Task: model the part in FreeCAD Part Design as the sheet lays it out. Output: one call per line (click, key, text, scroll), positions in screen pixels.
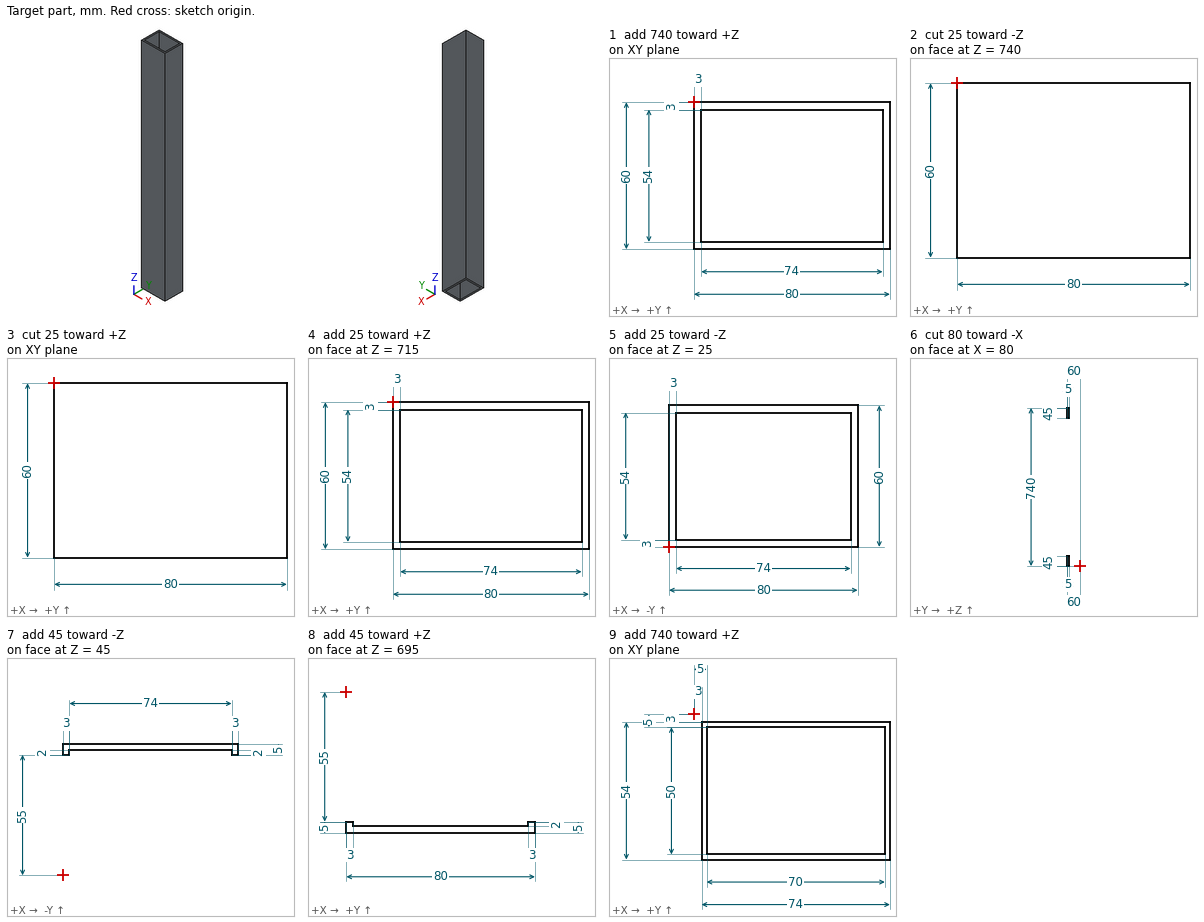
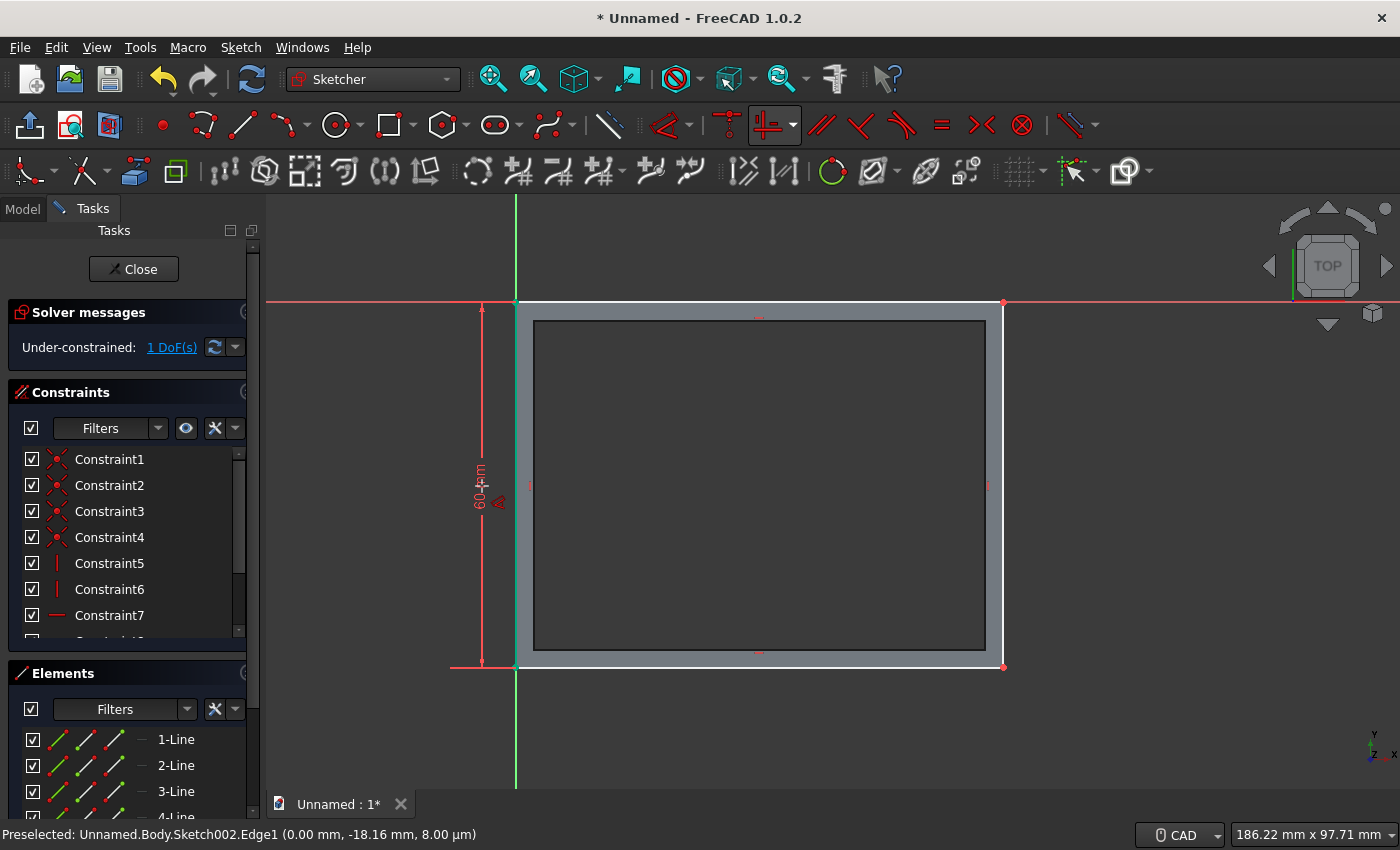
click(662, 668)
click(759, 702)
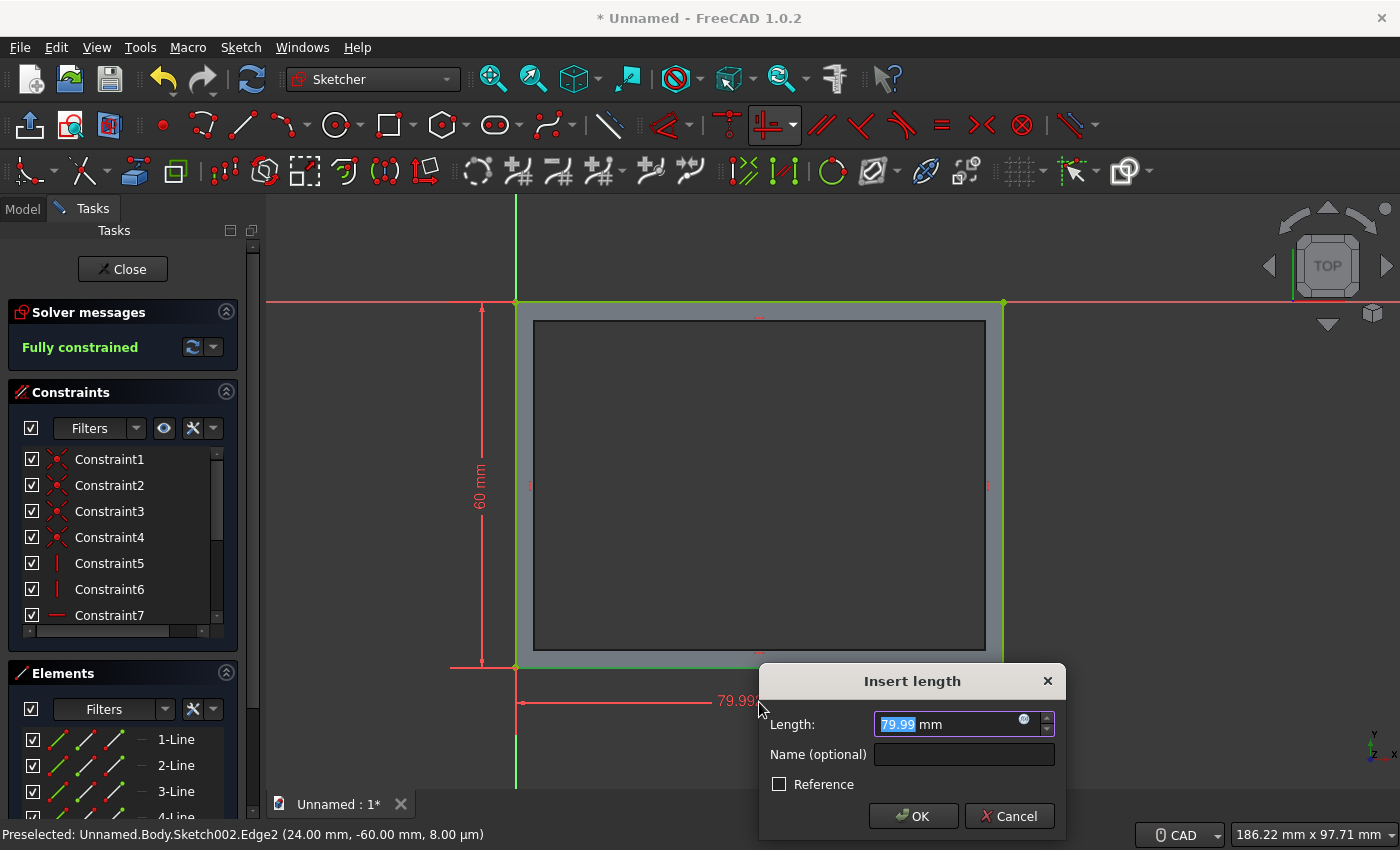
text(80)
key(Return)
key(Escape)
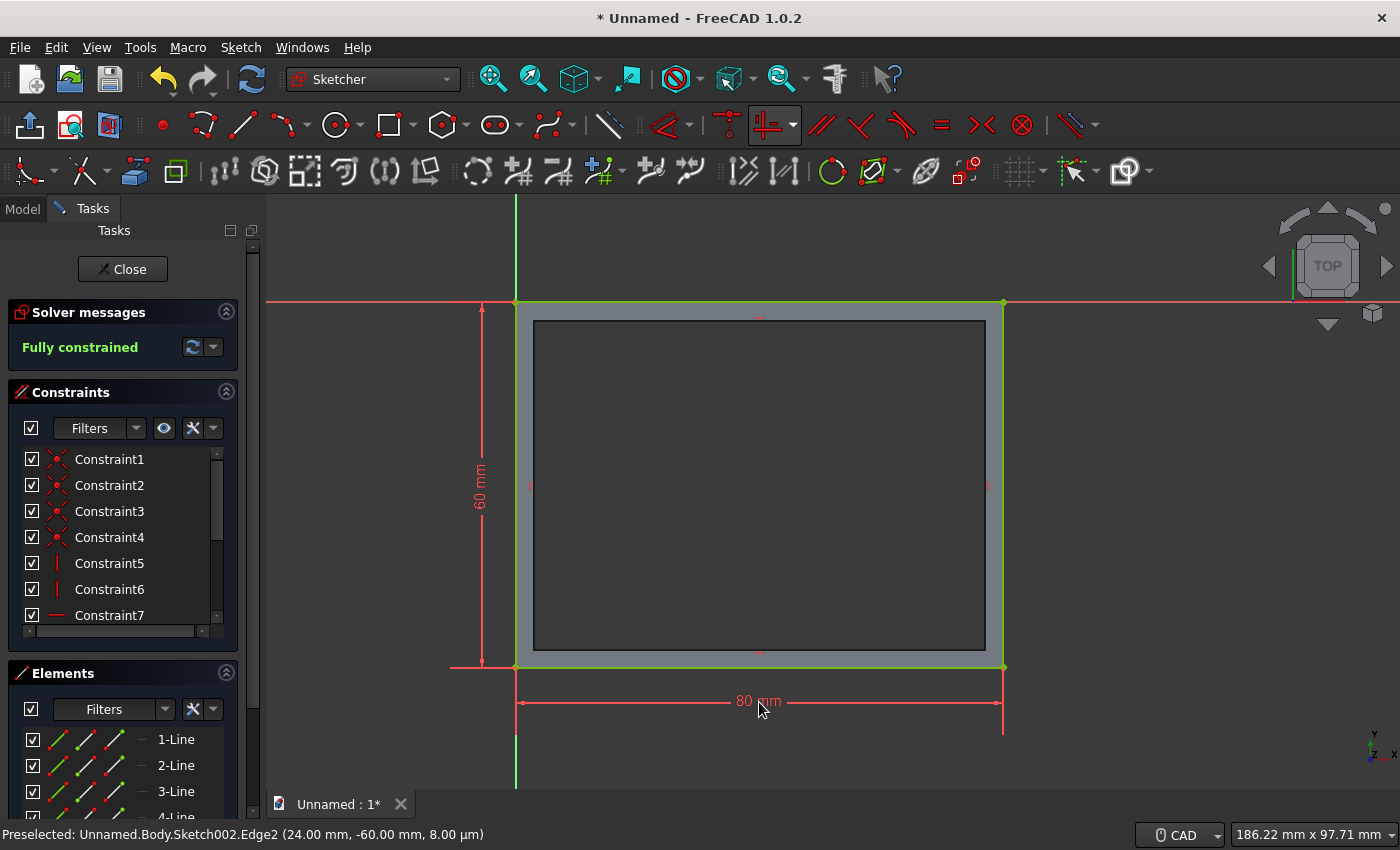
click(123, 269)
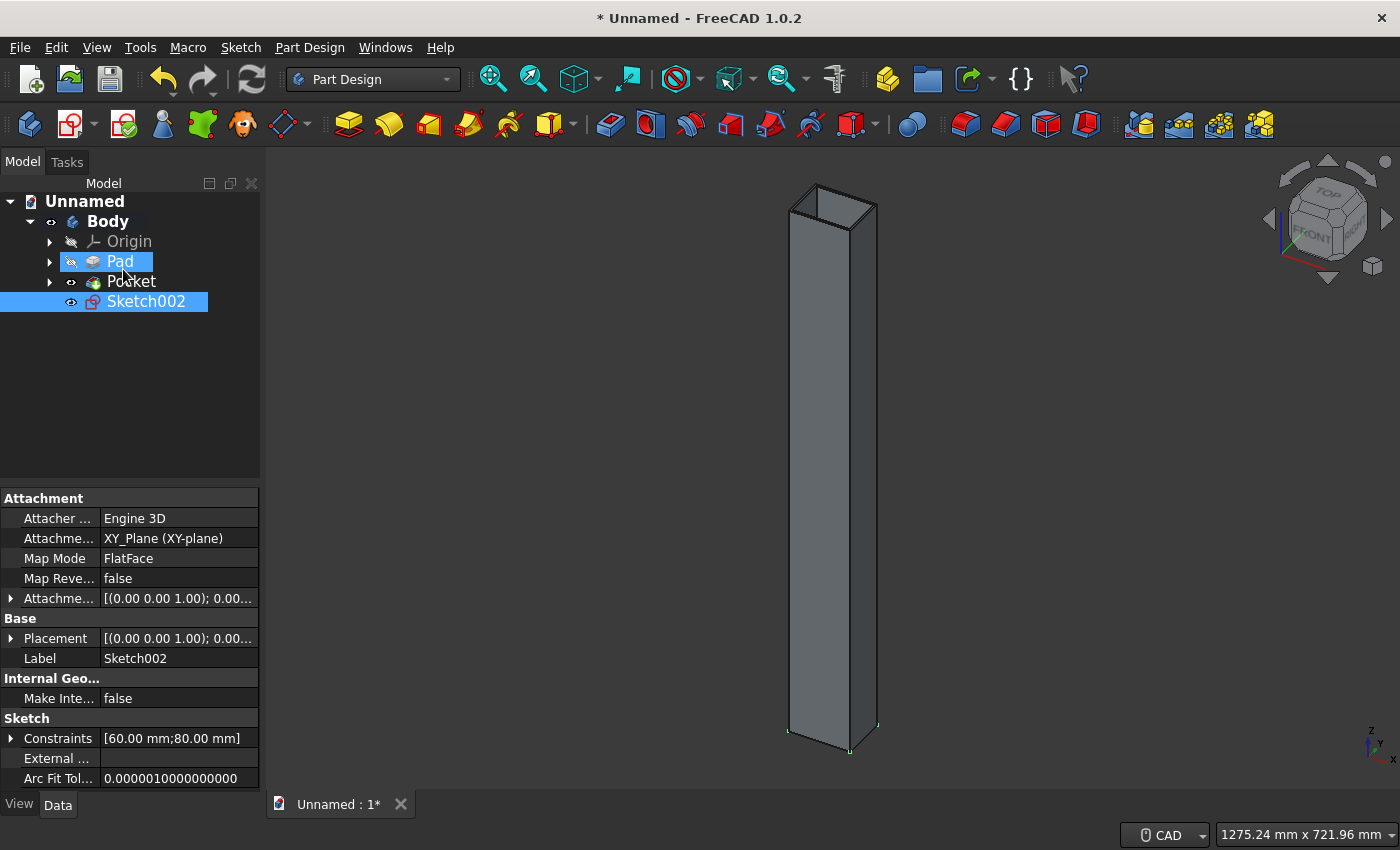
click(612, 124)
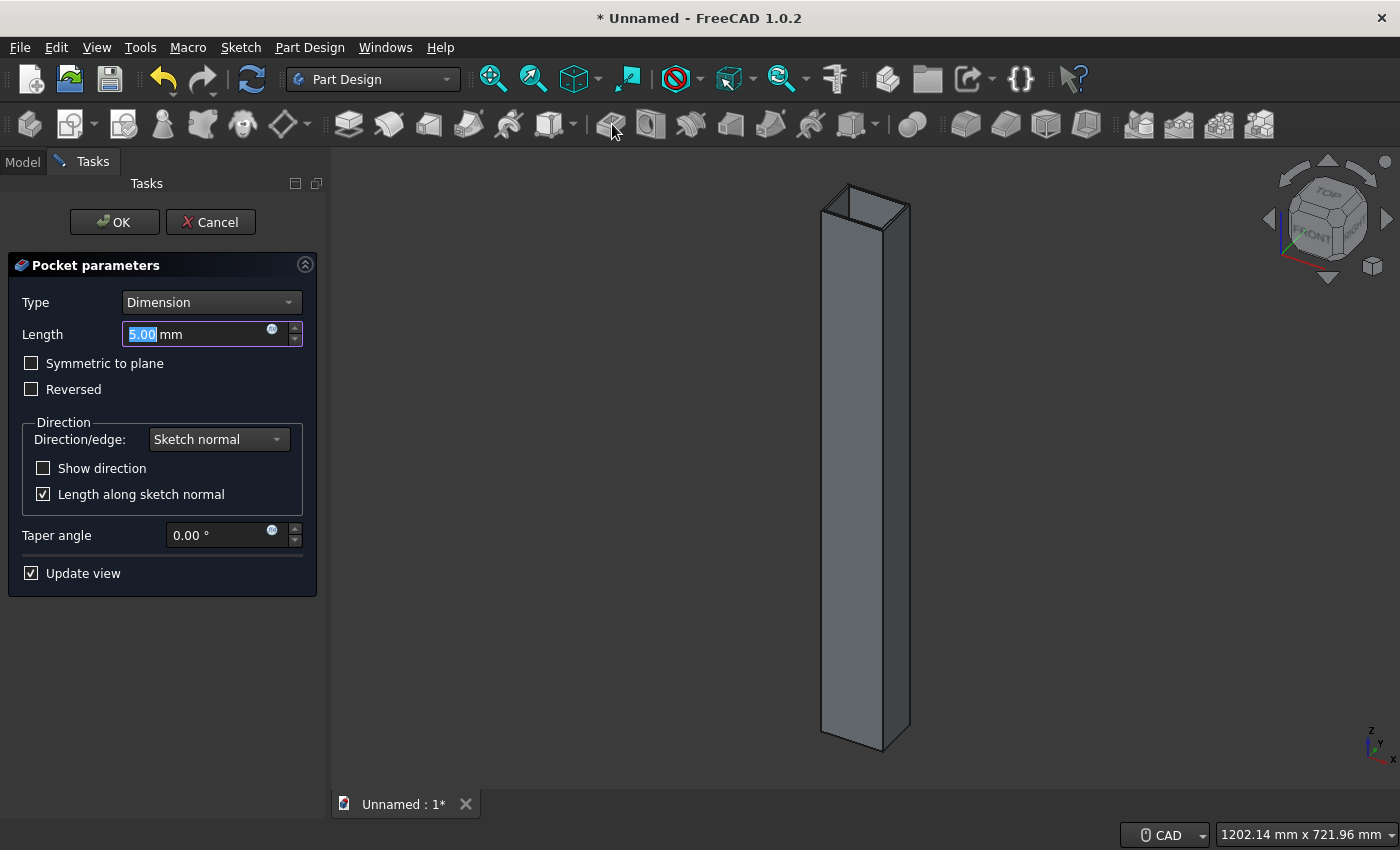
text(25)
key(Tab)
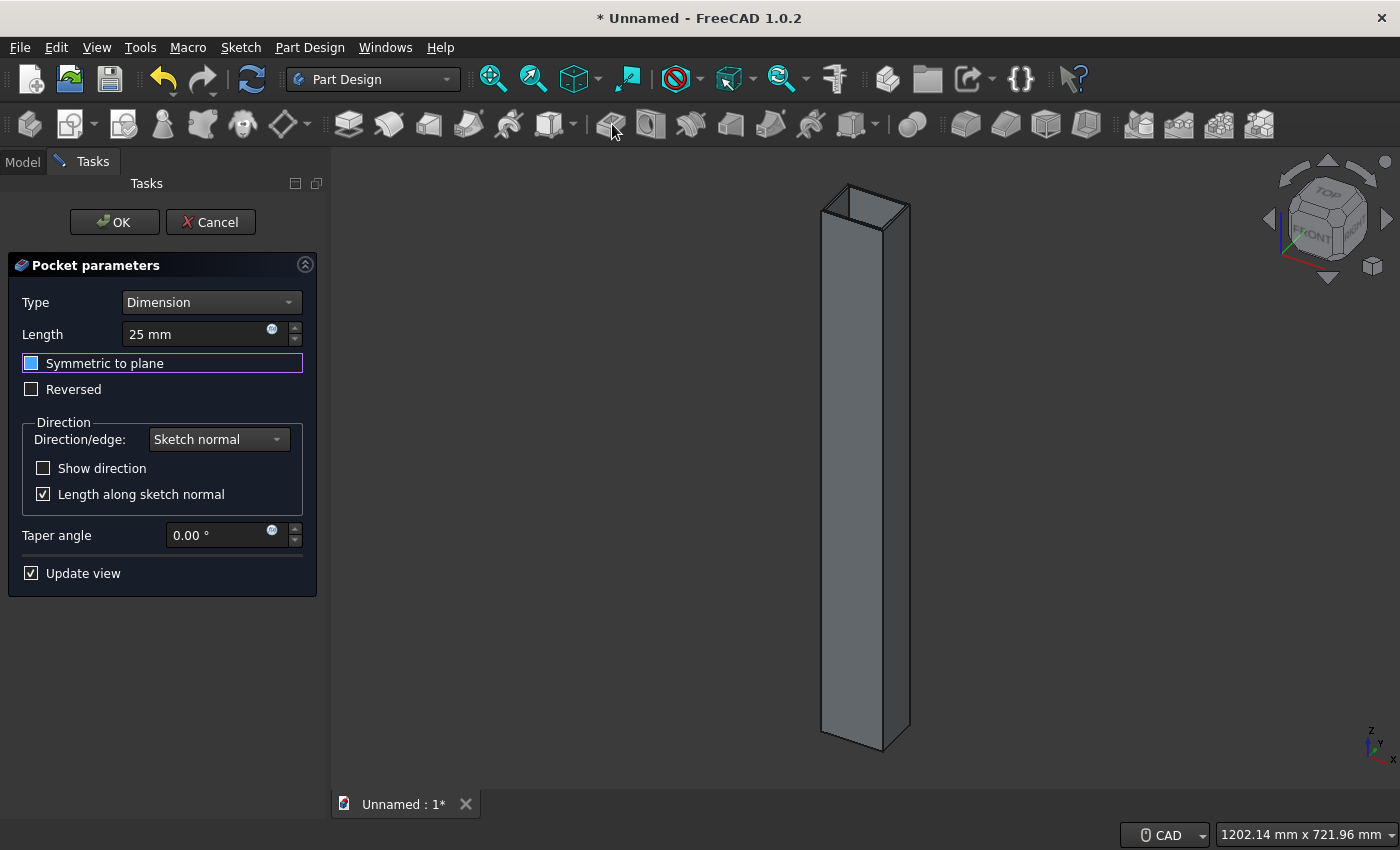
click(30, 389)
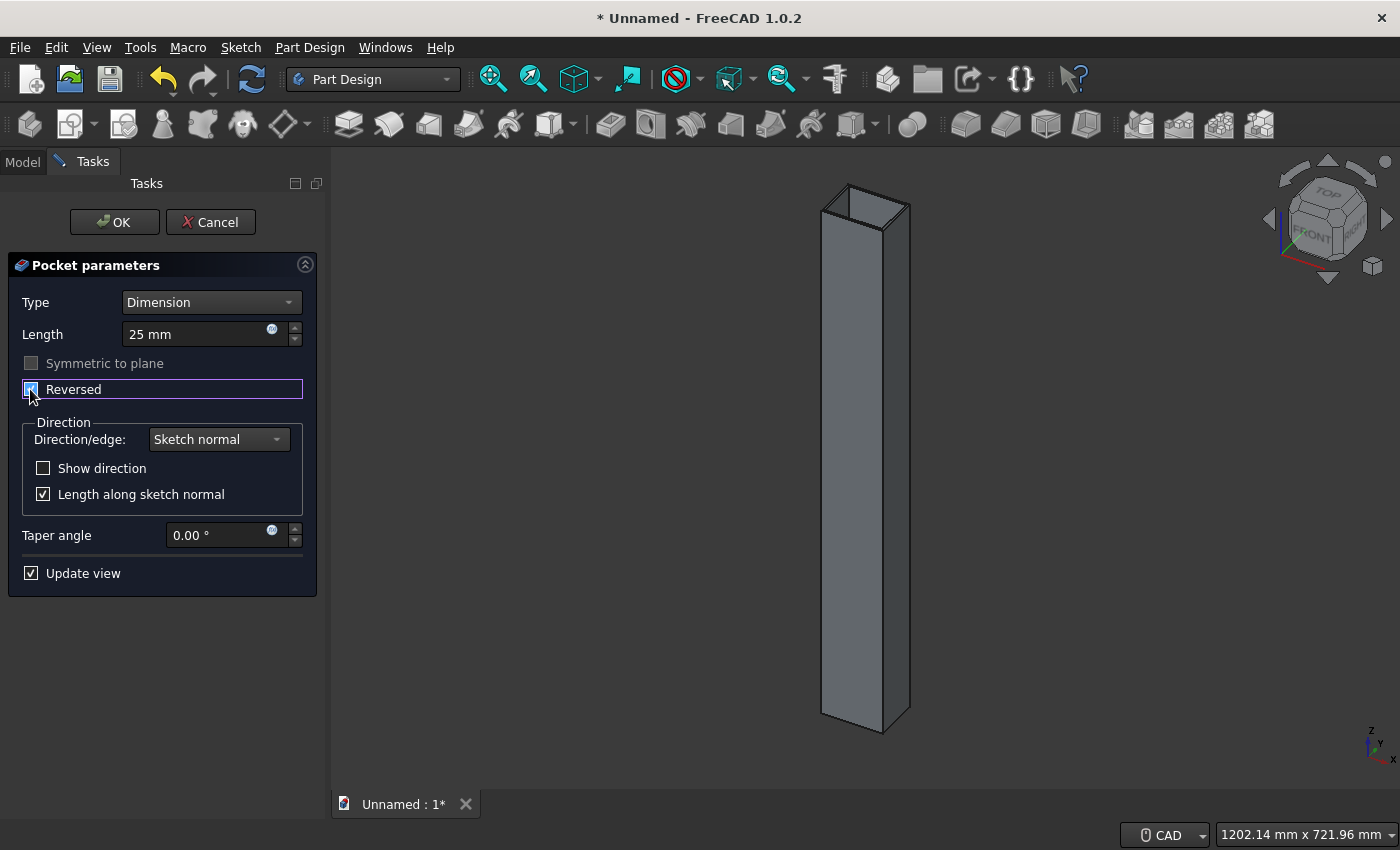
click(115, 222)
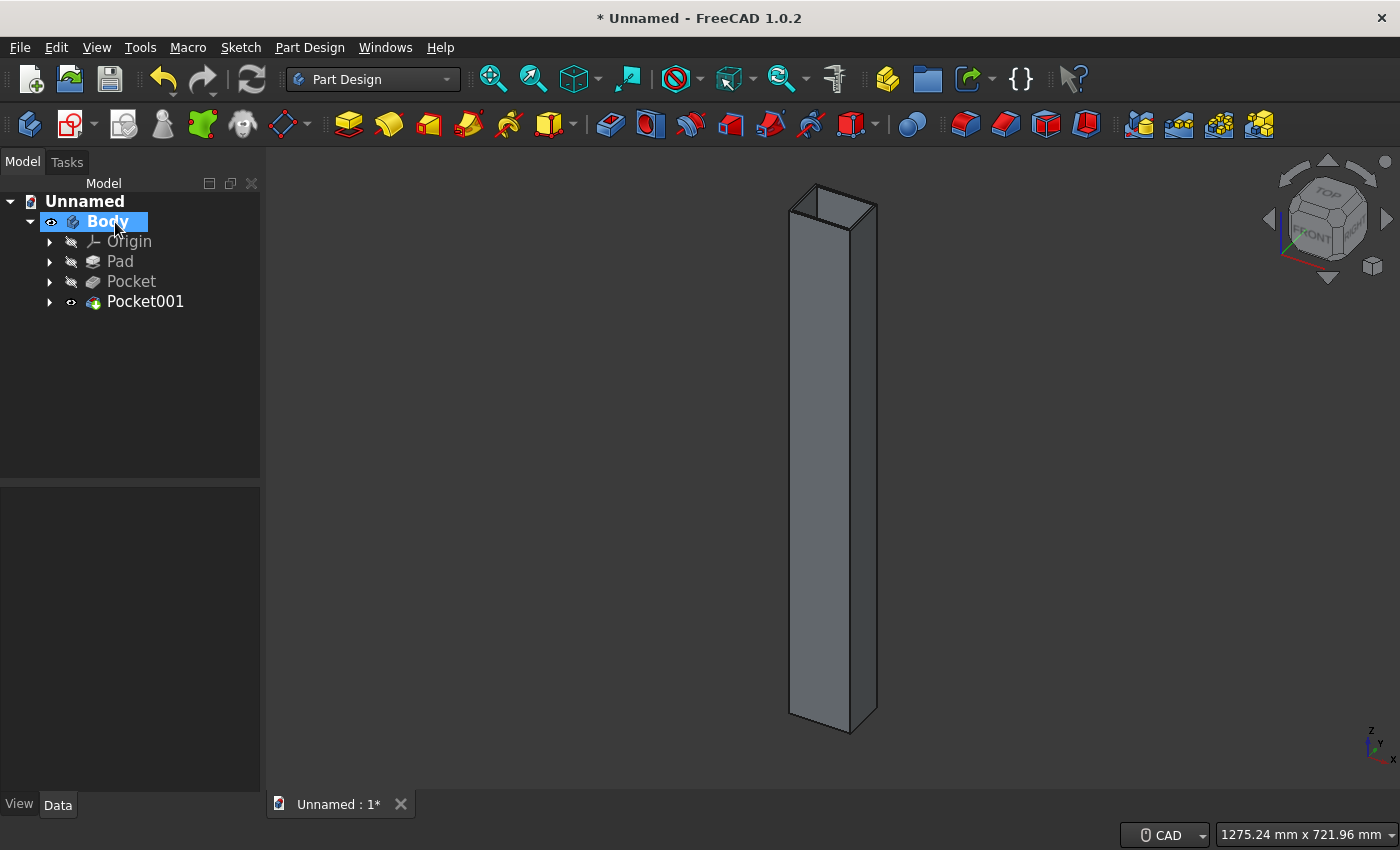
scroll(867, 213, up, 14)